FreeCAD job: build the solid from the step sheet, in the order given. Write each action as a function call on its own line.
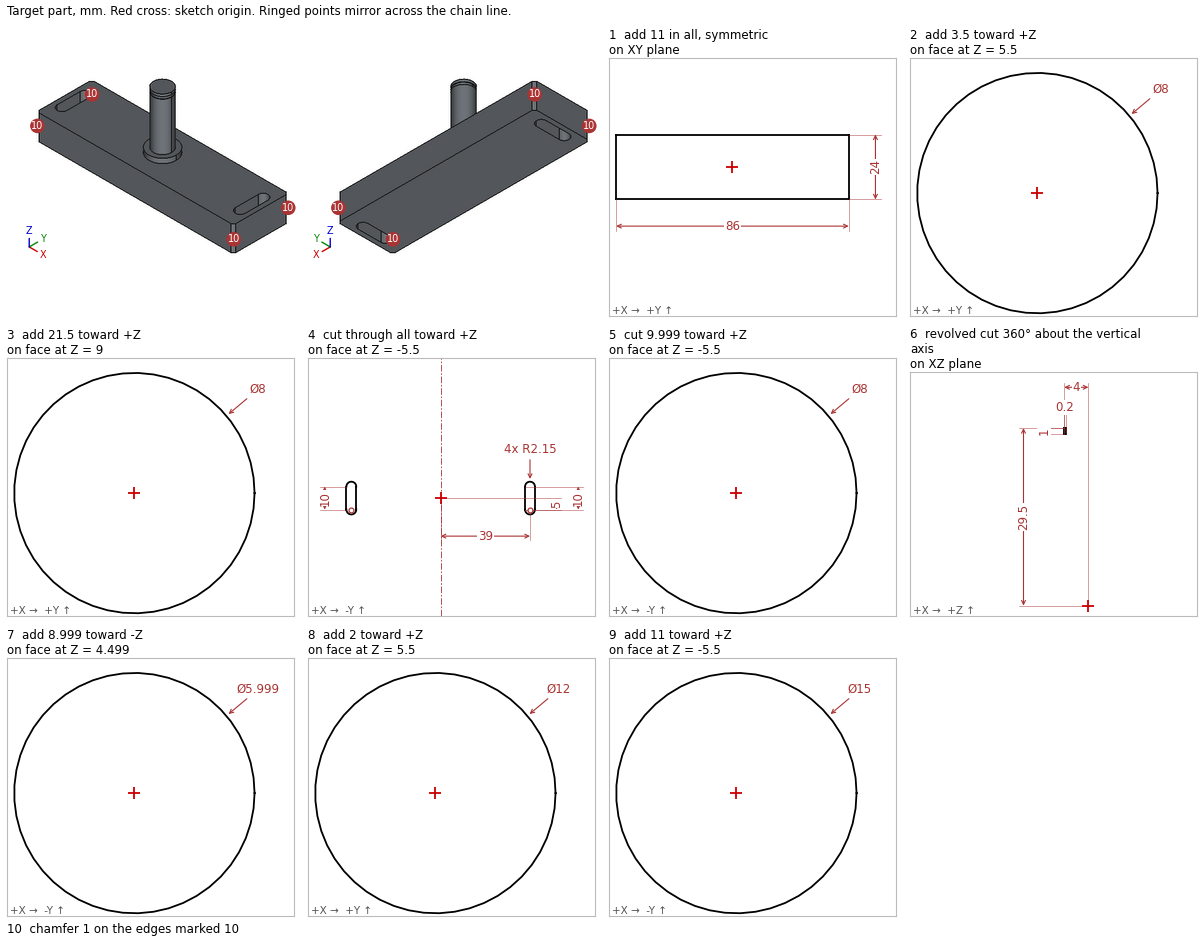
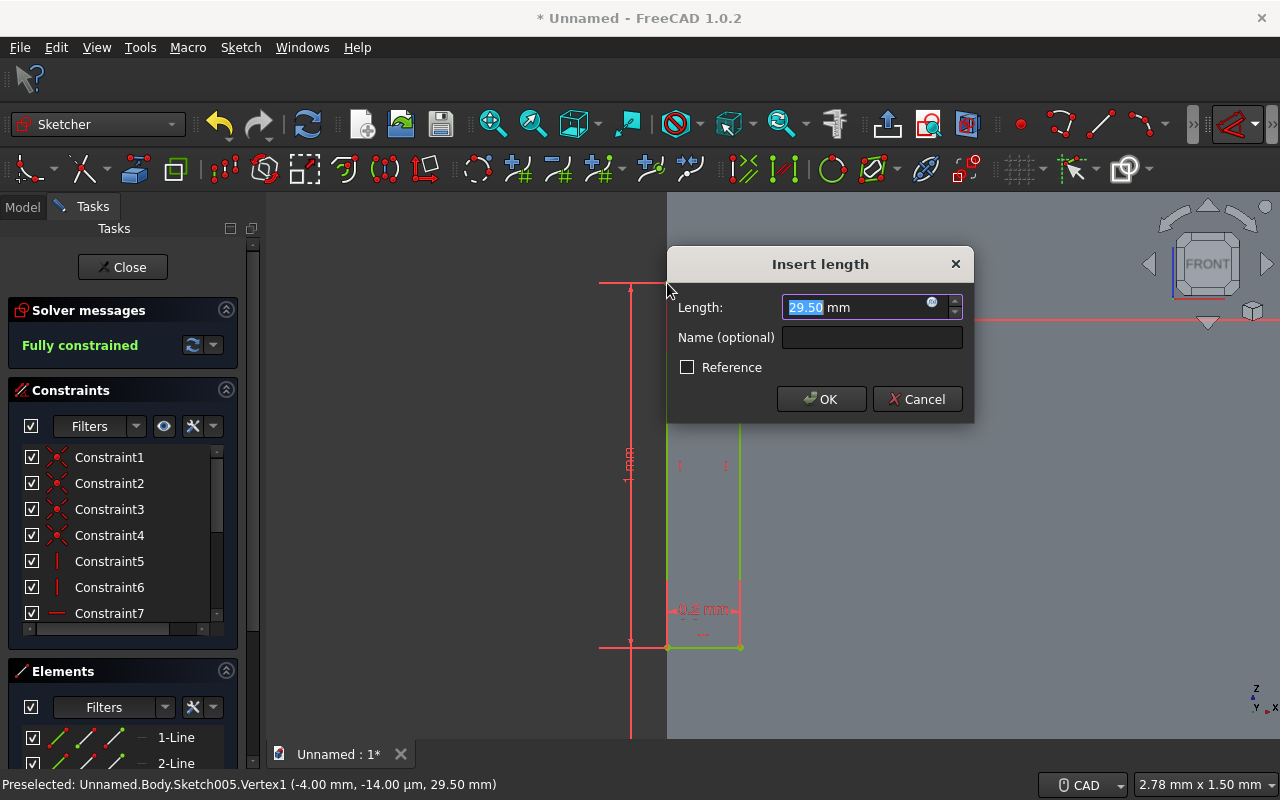
text(29.5)
key(Return)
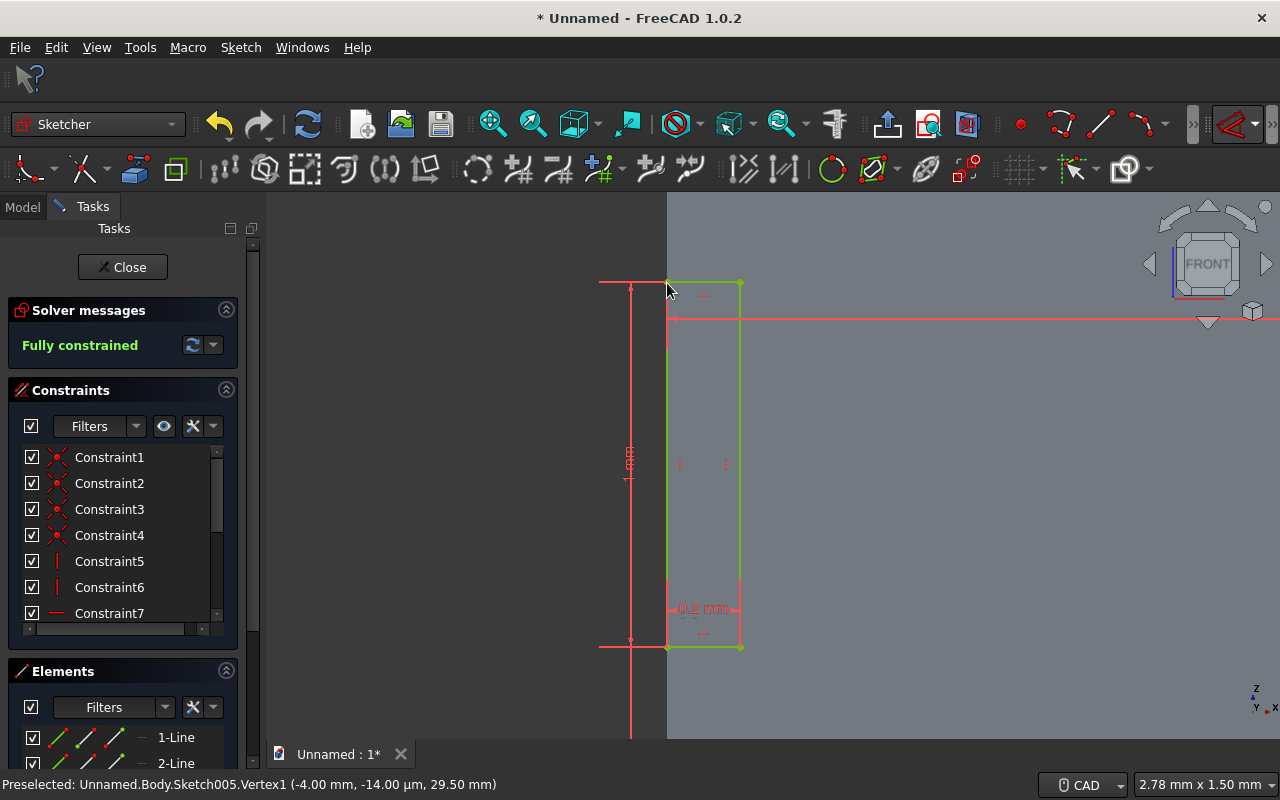
click(123, 267)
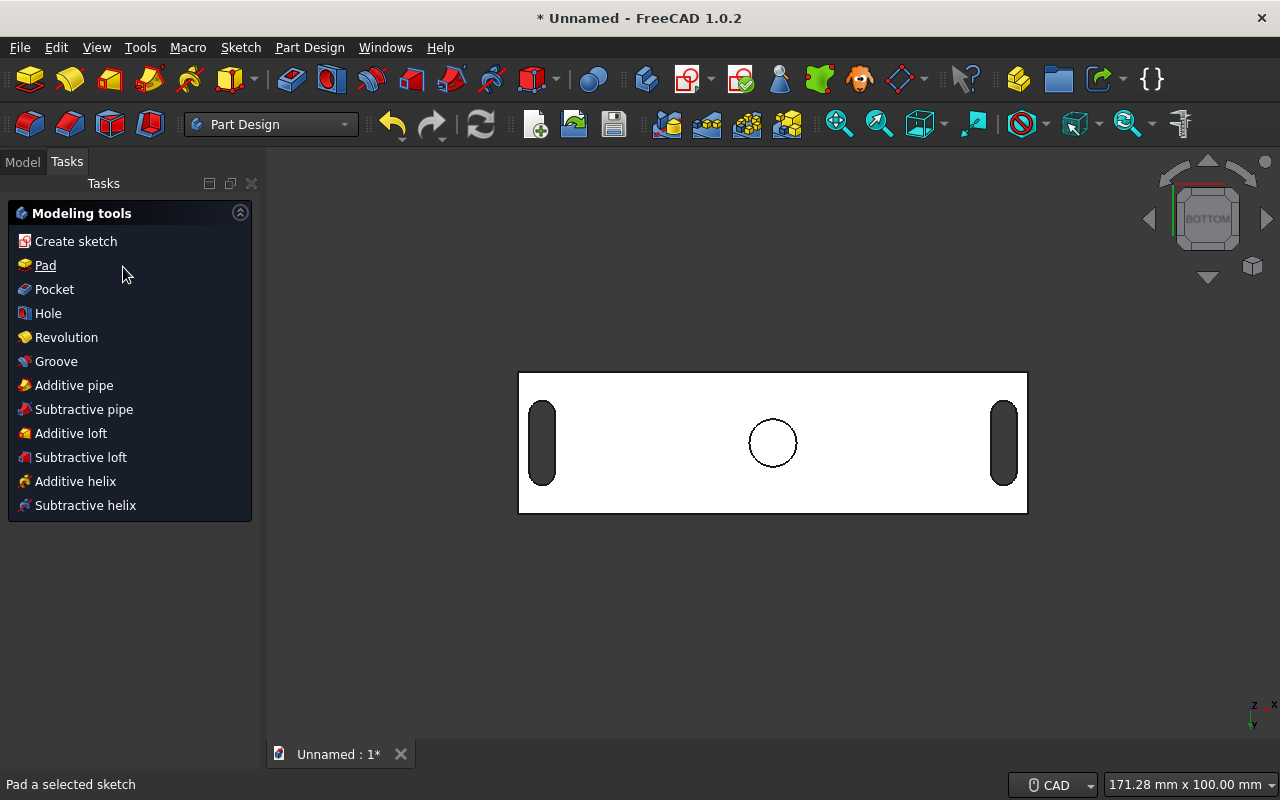
click(372, 80)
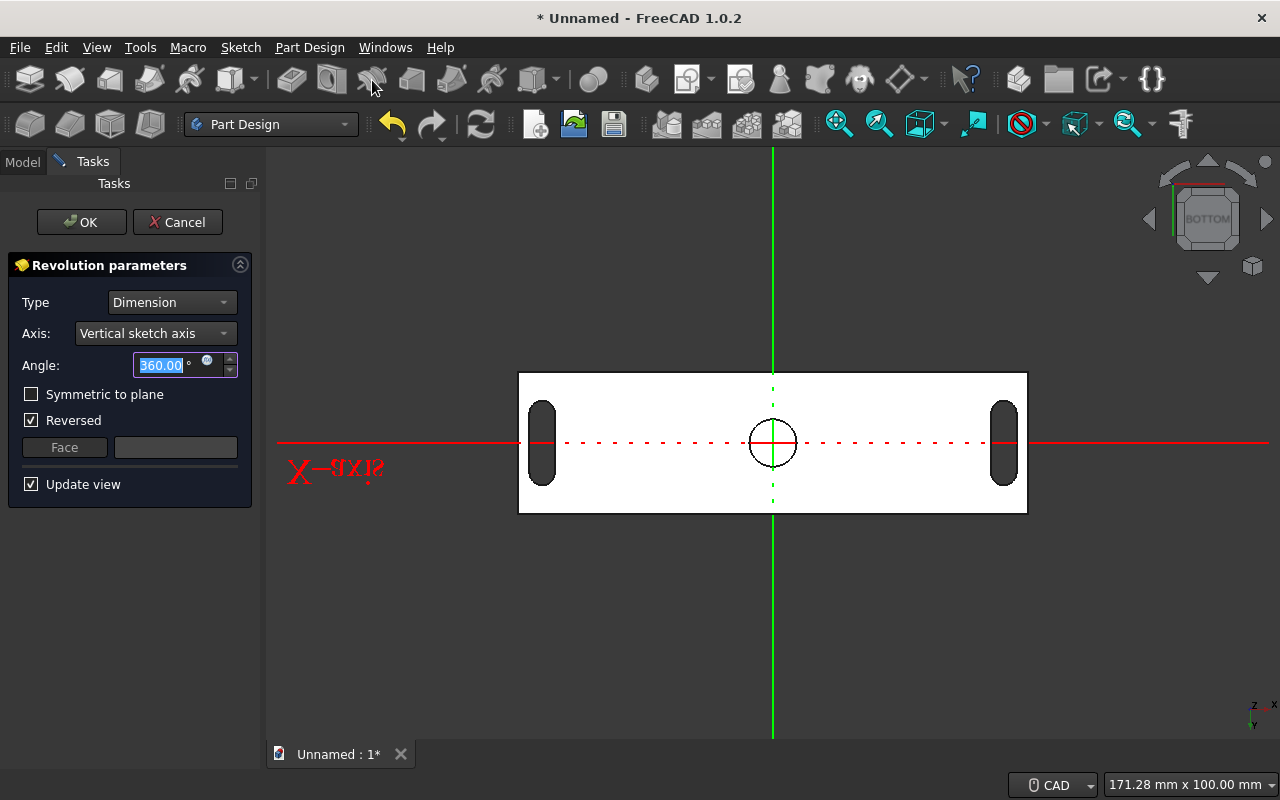
click(82, 222)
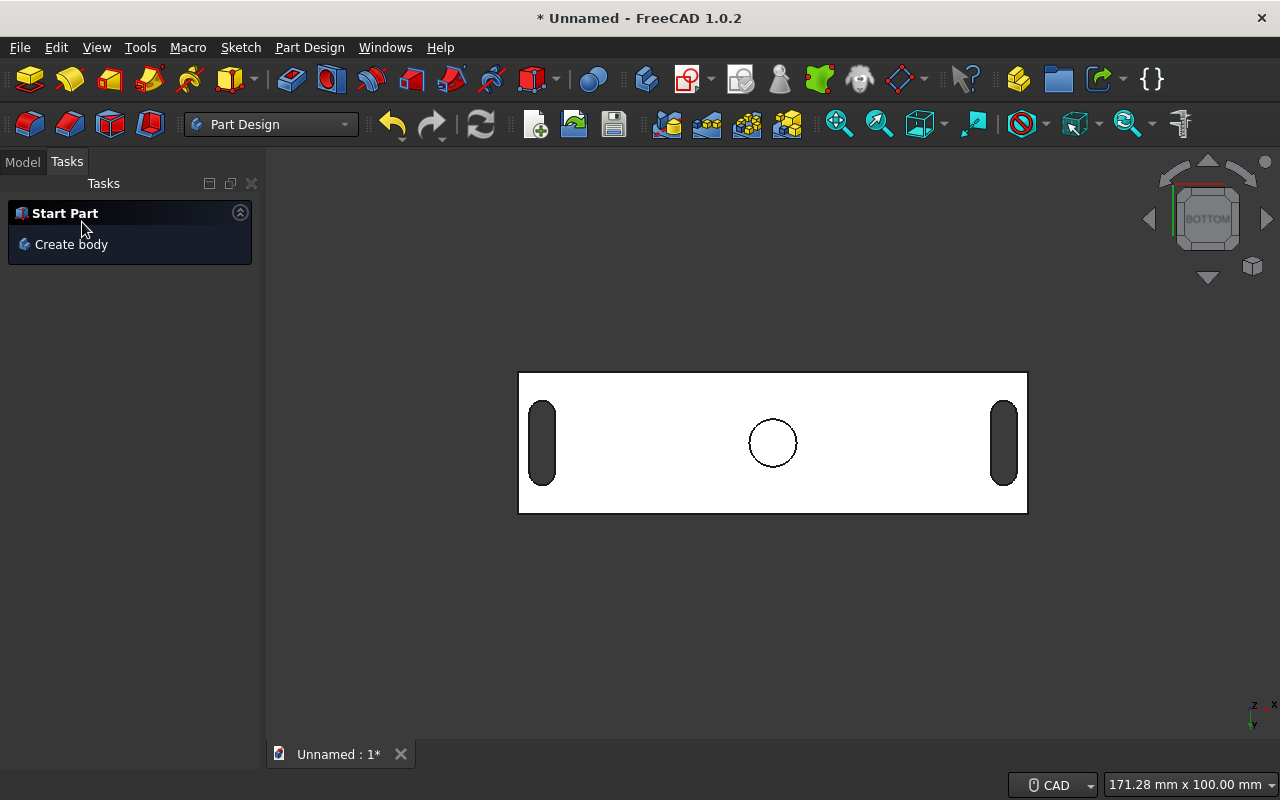
click(773, 442)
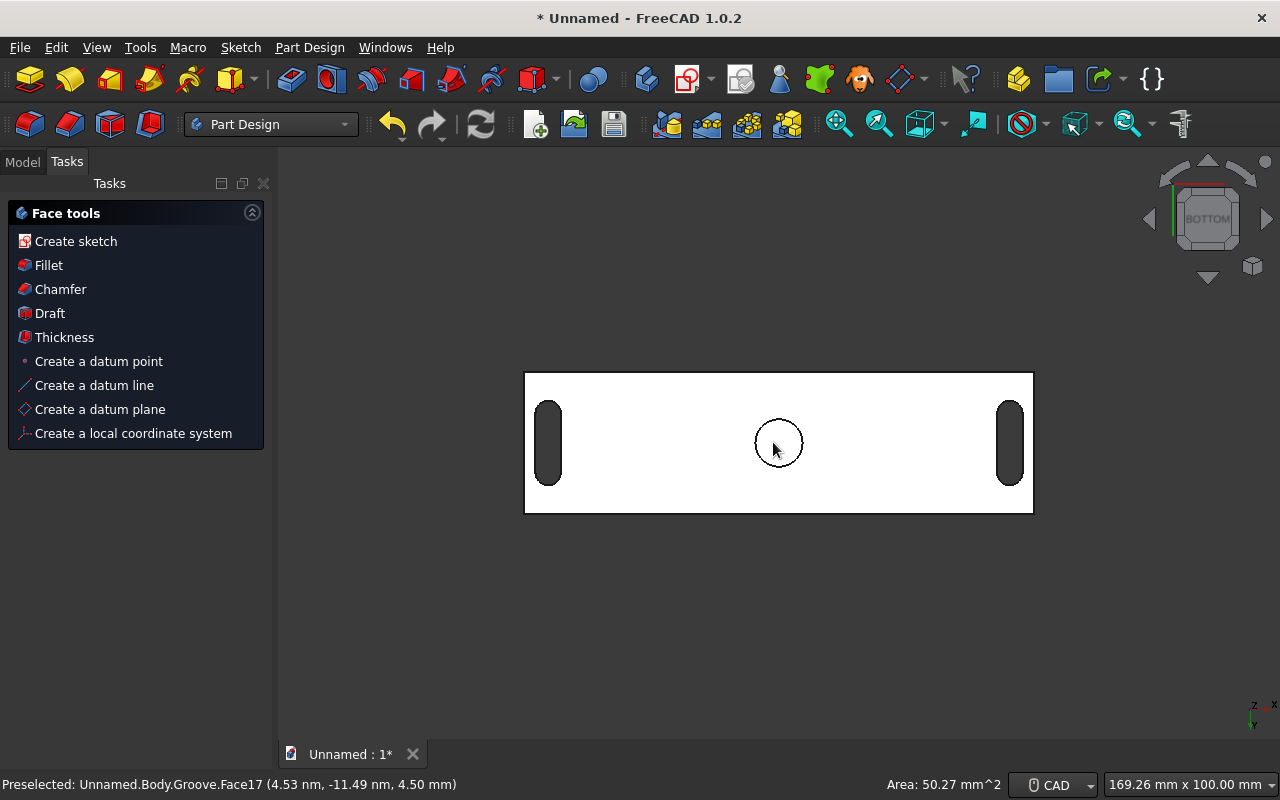
click(688, 80)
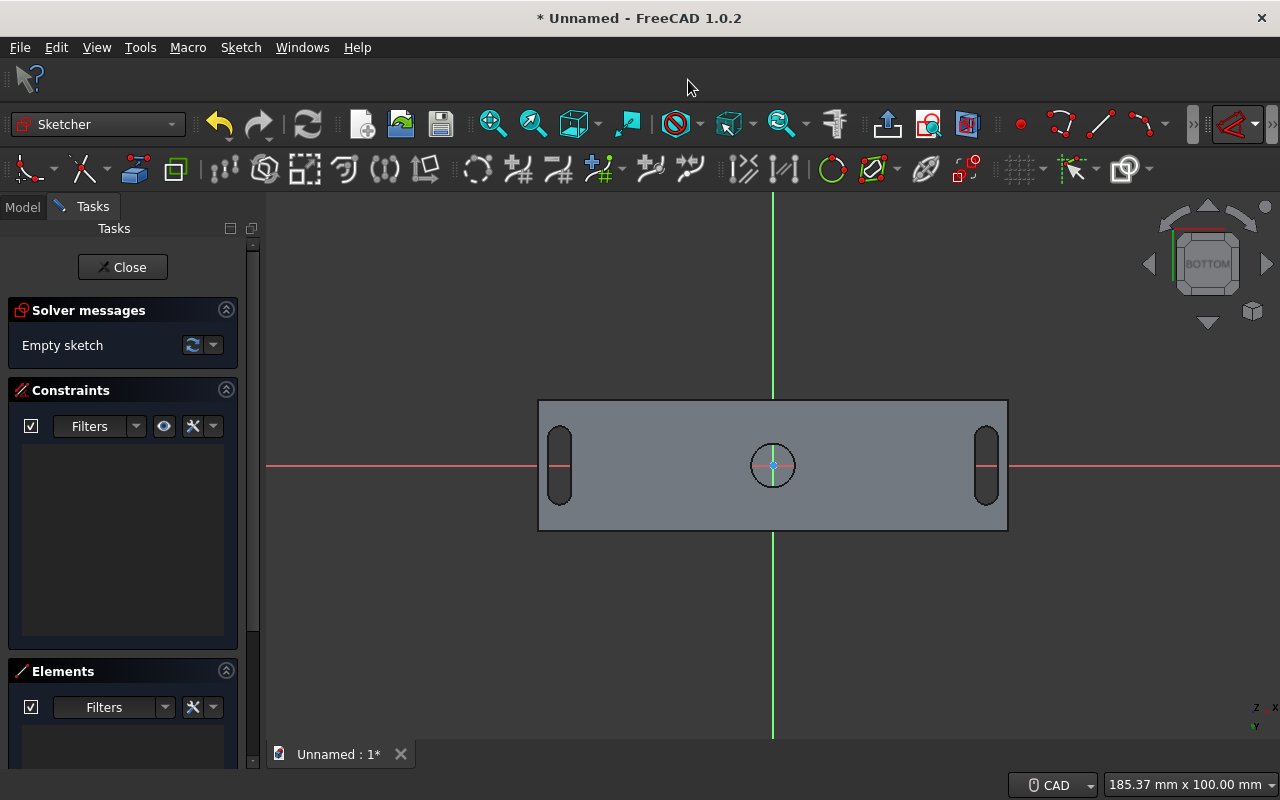
click(968, 124)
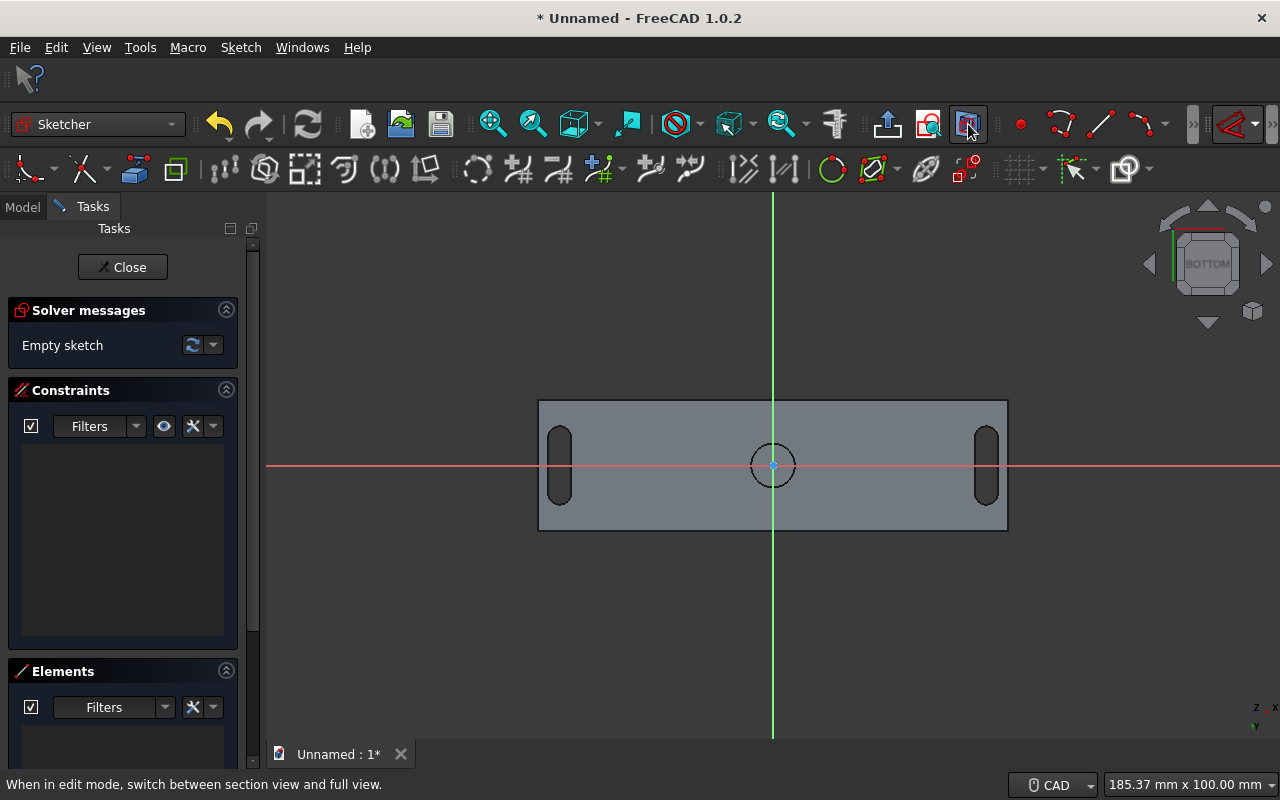
scroll(780, 466, up, 12)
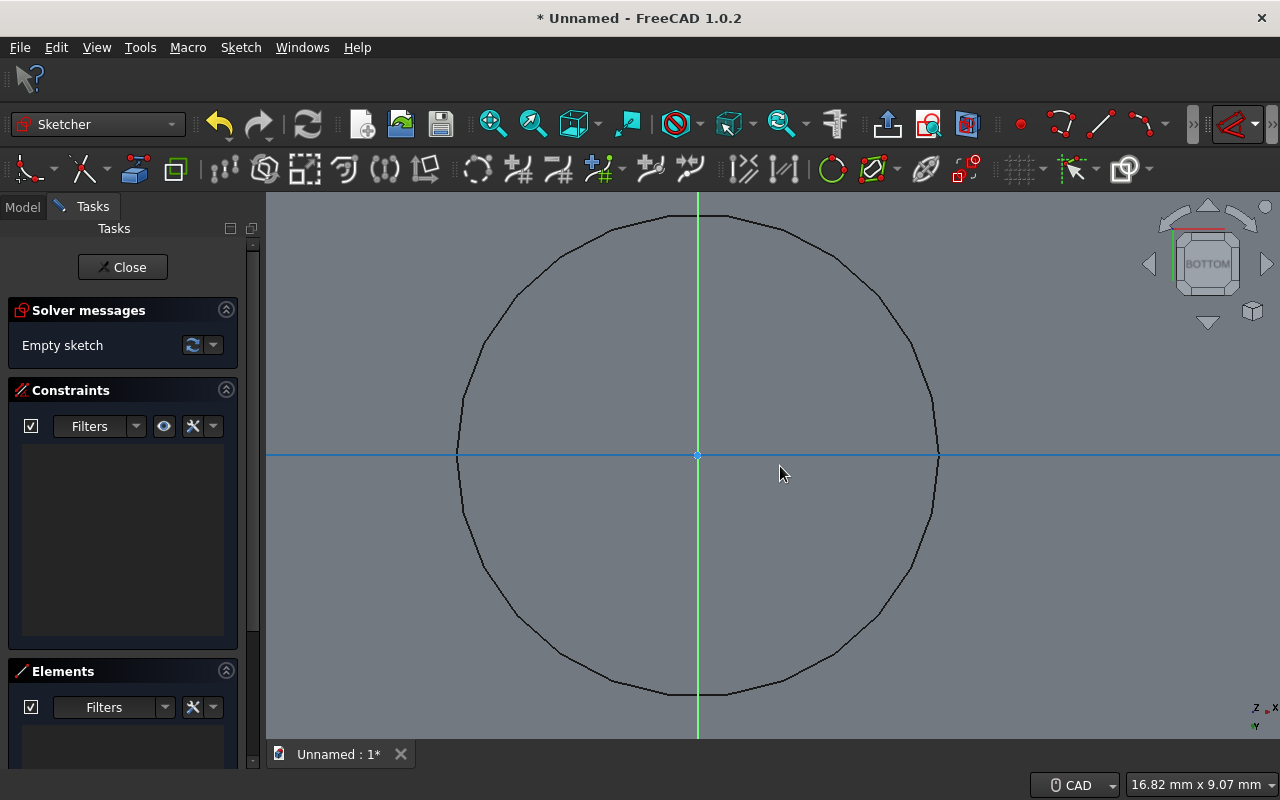
key(g)
key(c)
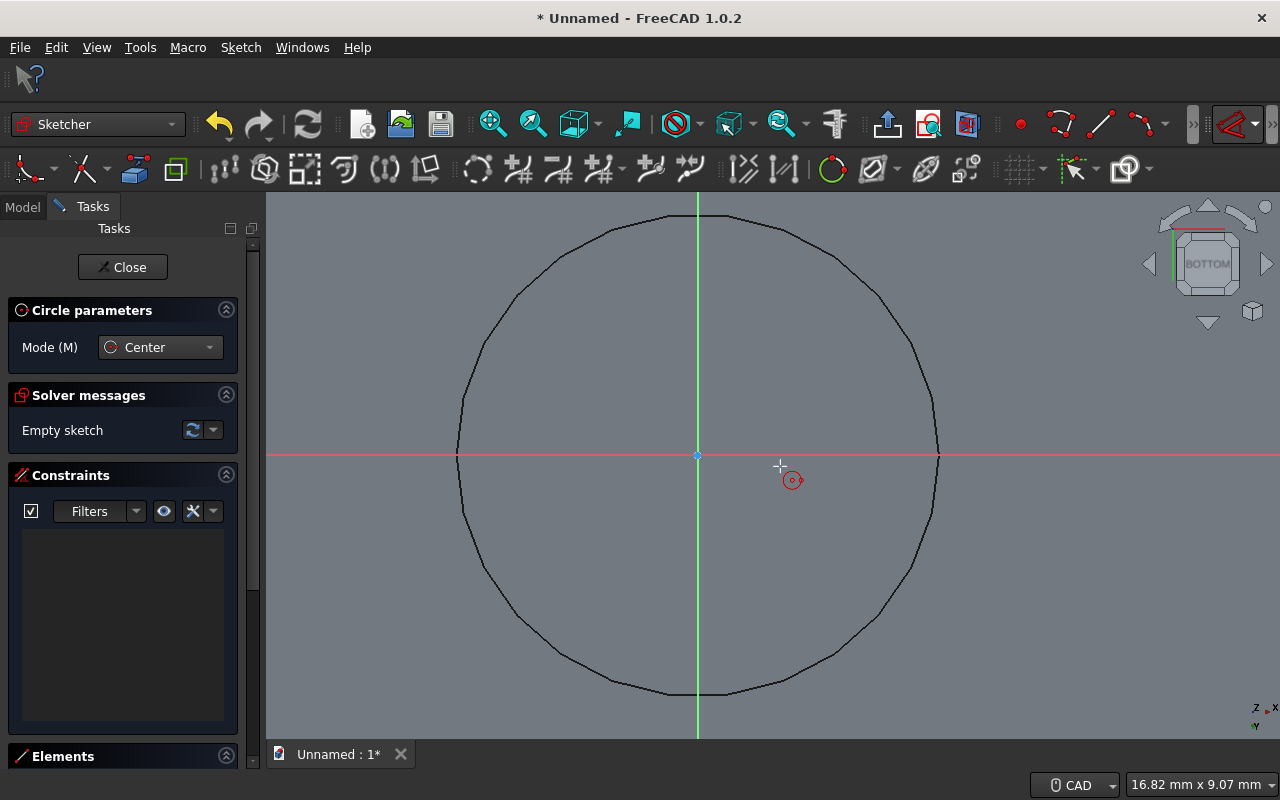
click(698, 455)
move(826, 328)